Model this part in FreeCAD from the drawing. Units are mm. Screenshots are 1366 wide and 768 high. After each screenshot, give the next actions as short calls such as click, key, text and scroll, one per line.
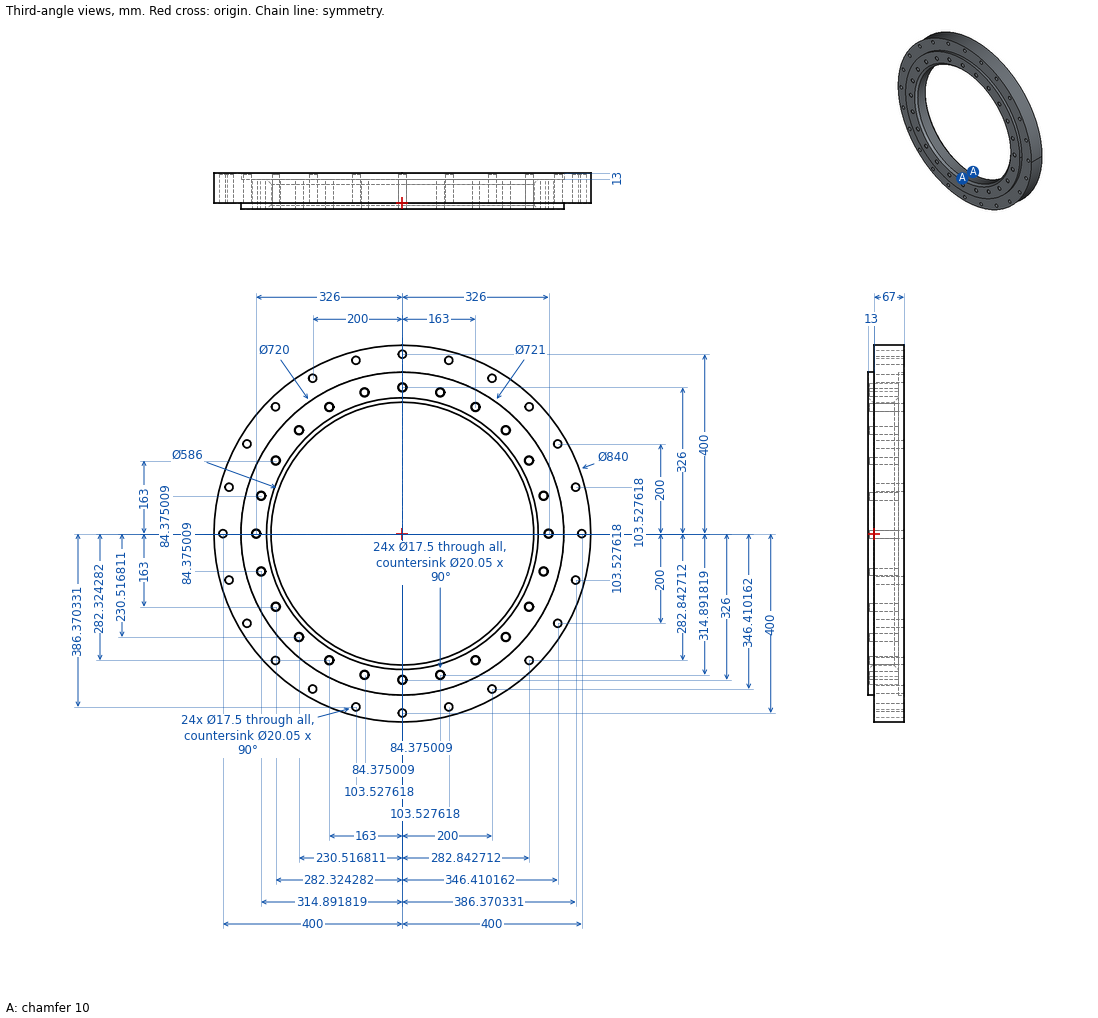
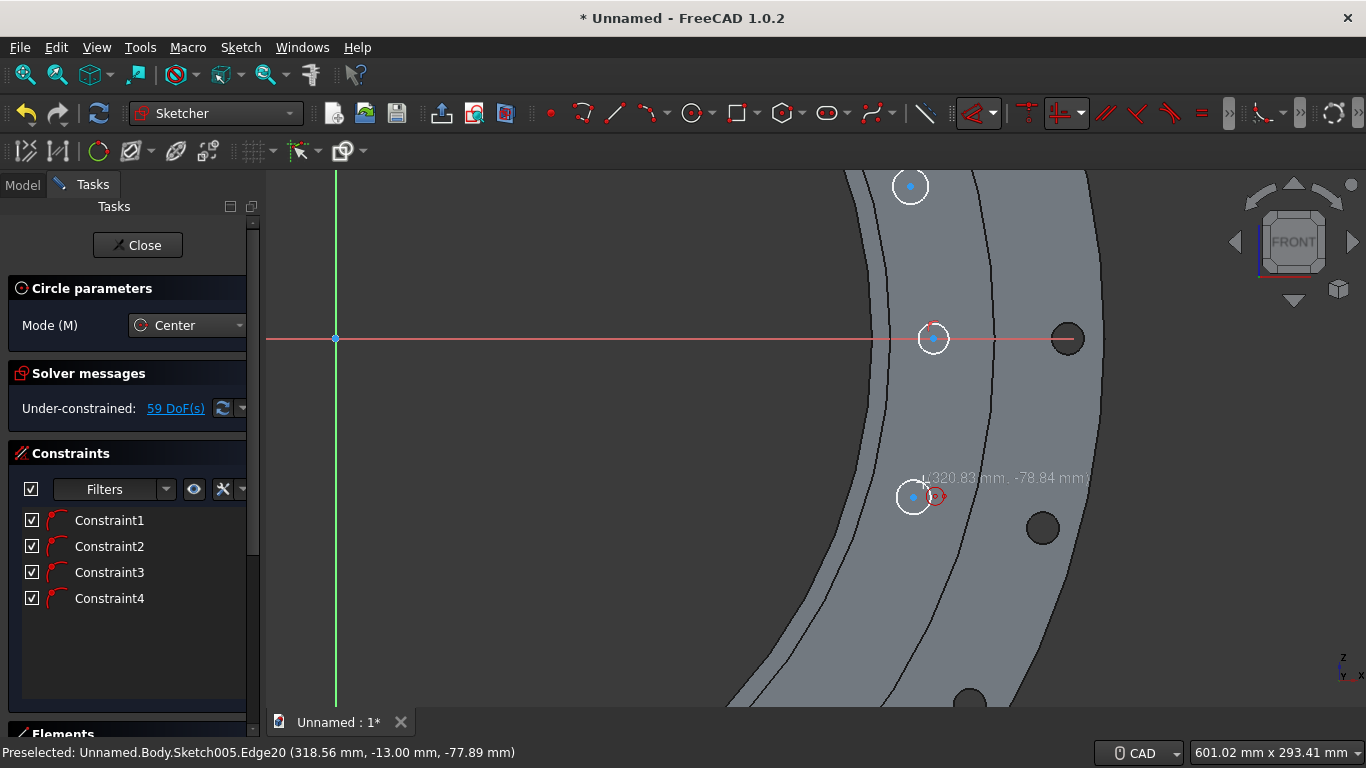
scroll(853, 637, up, 2)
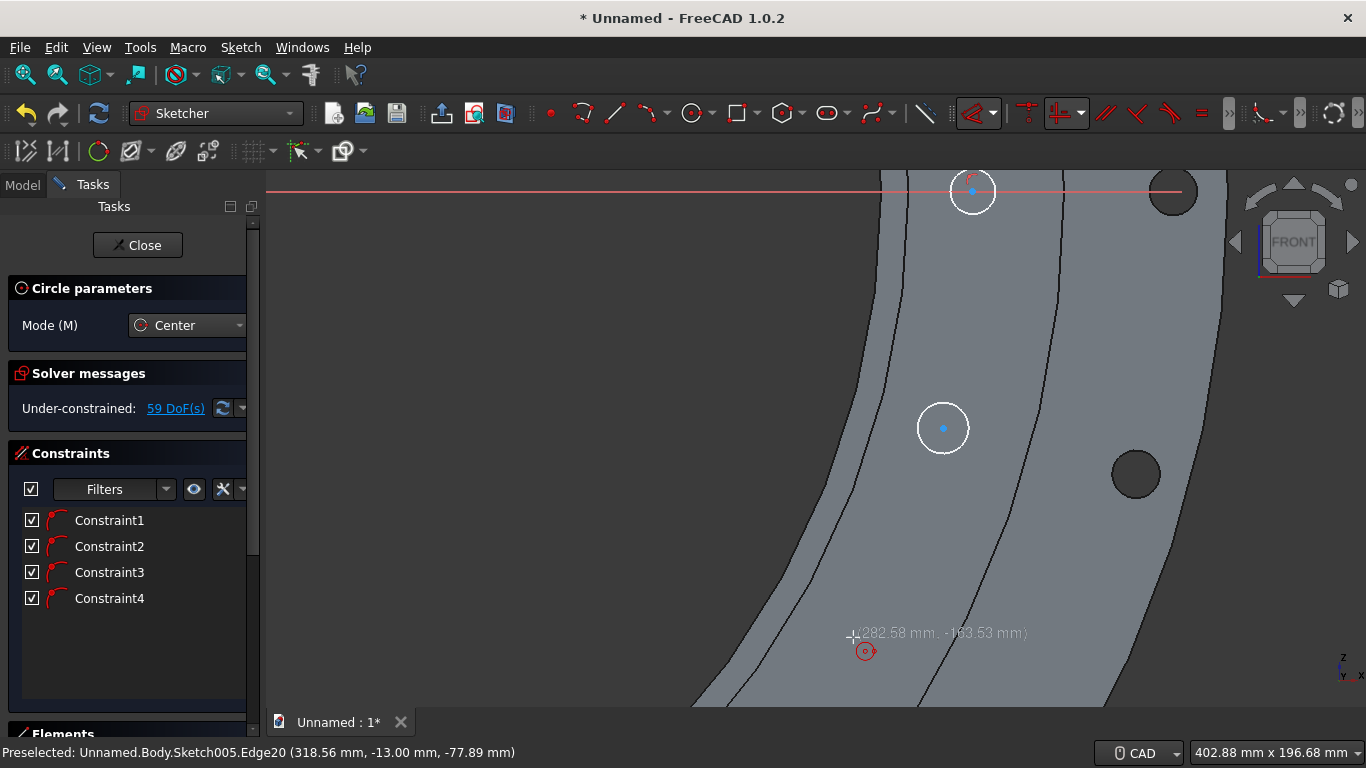
scroll(916, 501, down, 8)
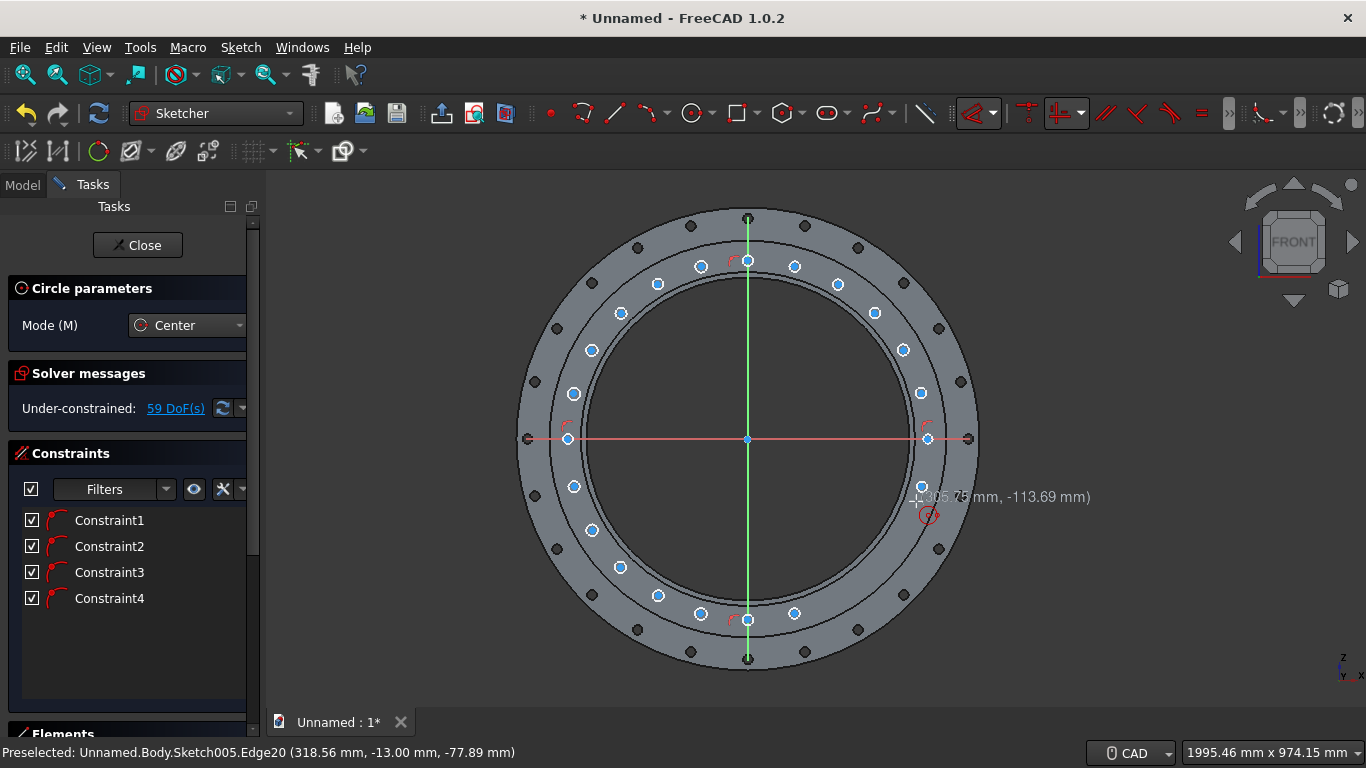
click(904, 529)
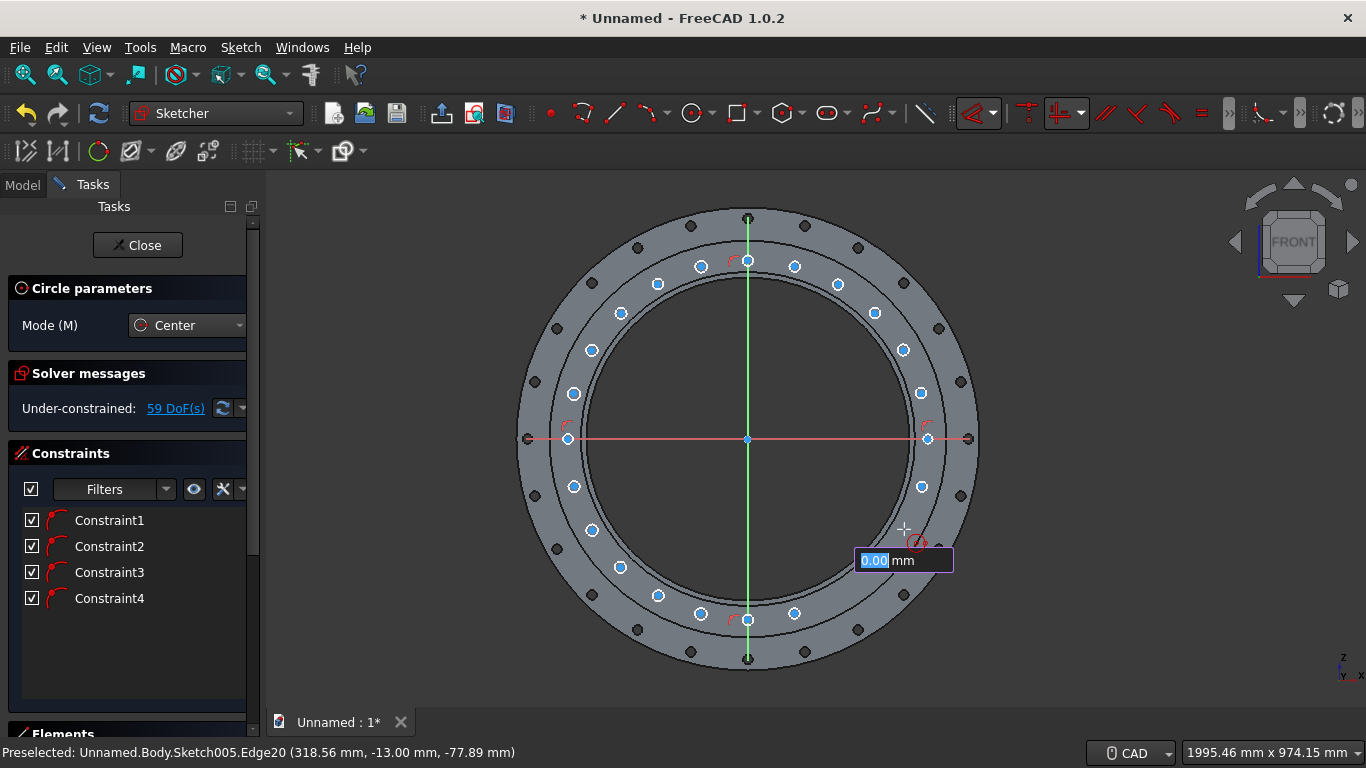
scroll(907, 525, up, 6)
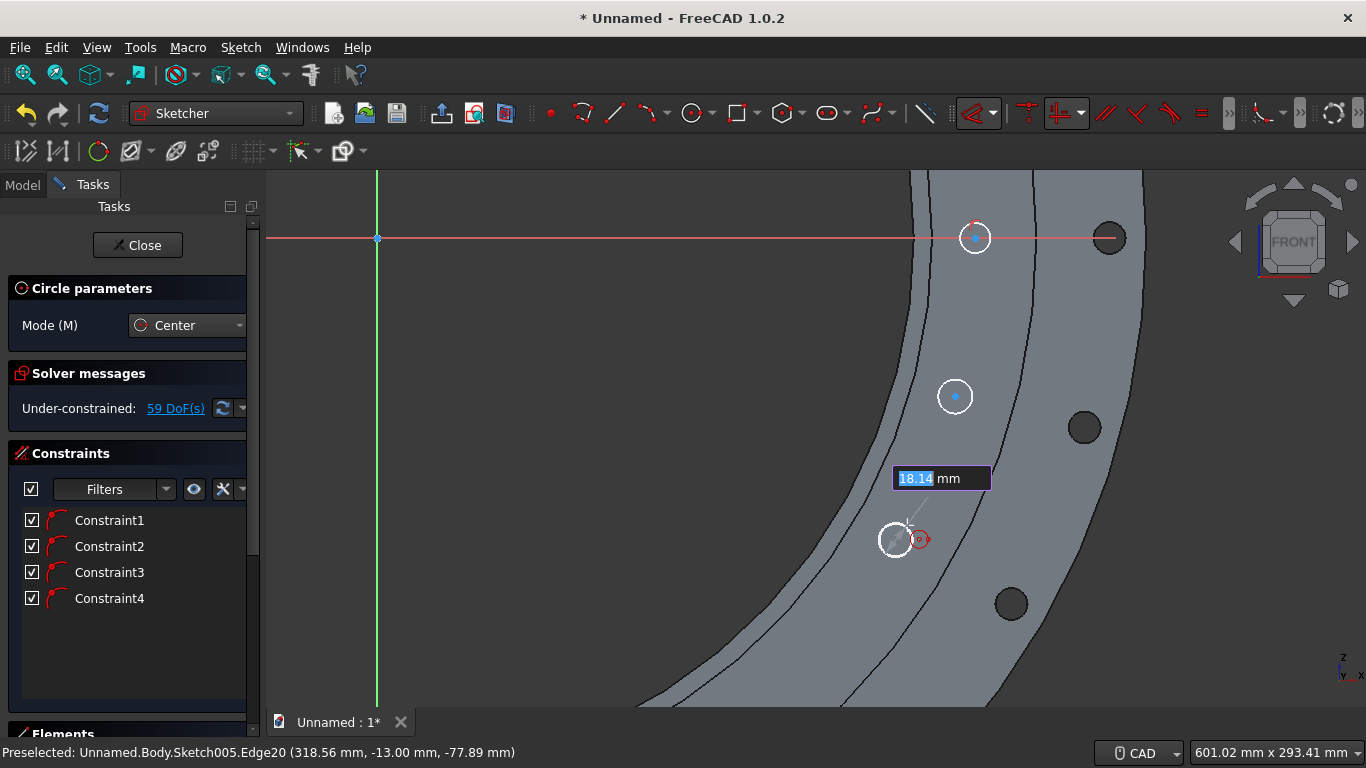
click(906, 525)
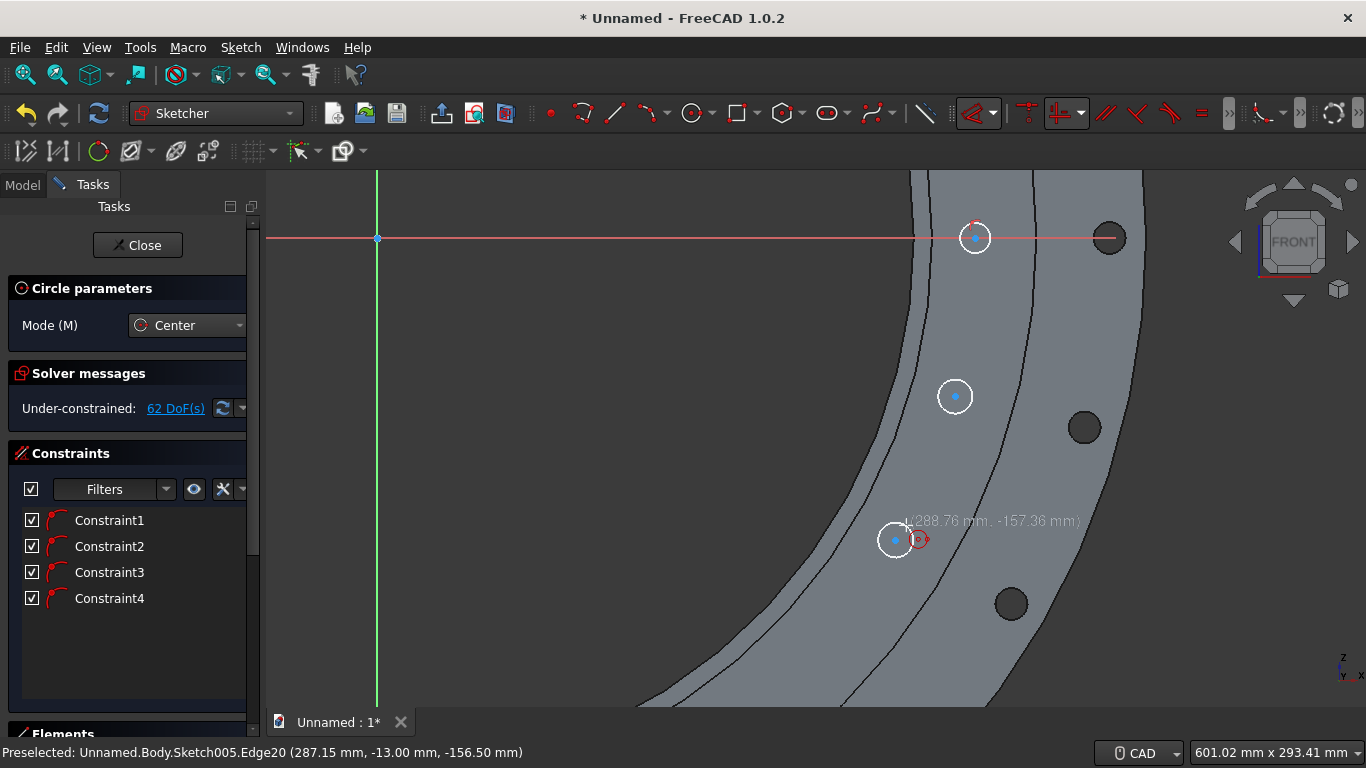
scroll(799, 660, up, 2)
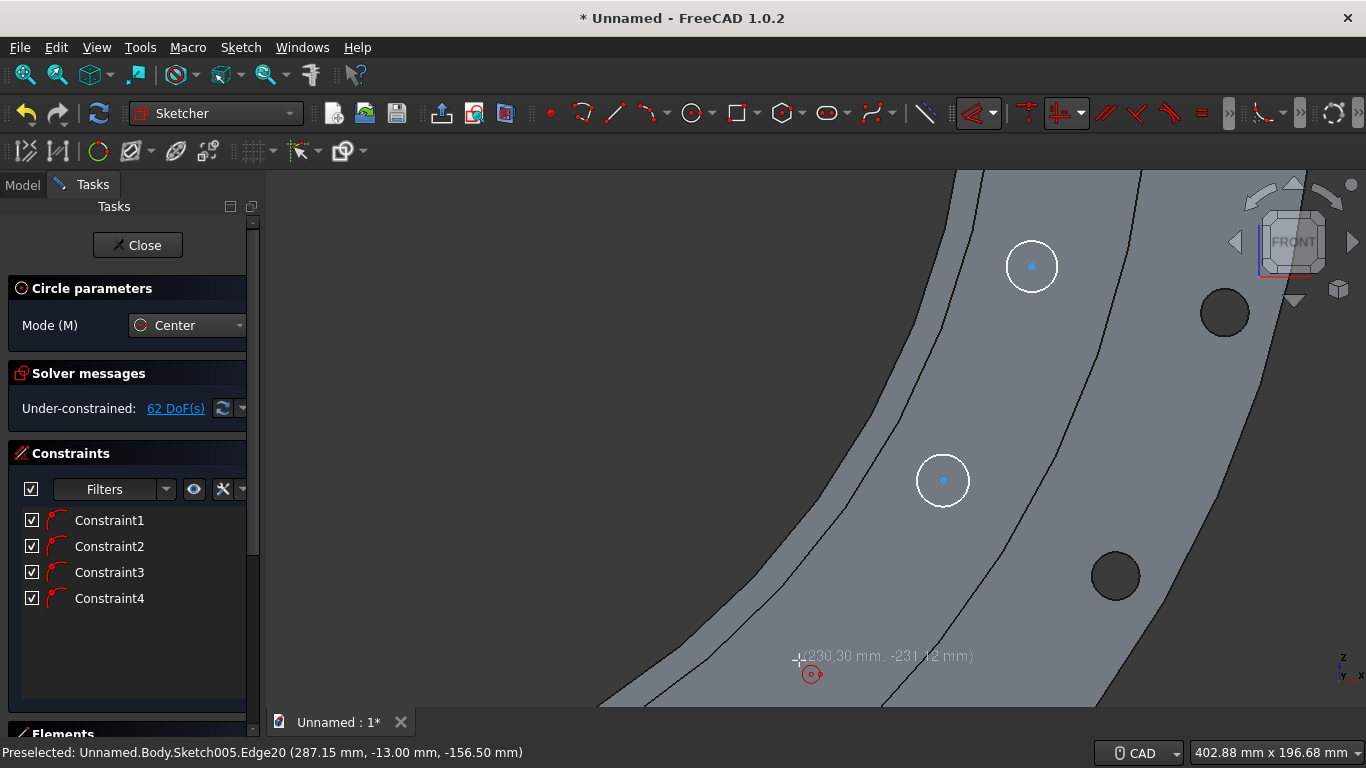
scroll(894, 542, down, 8)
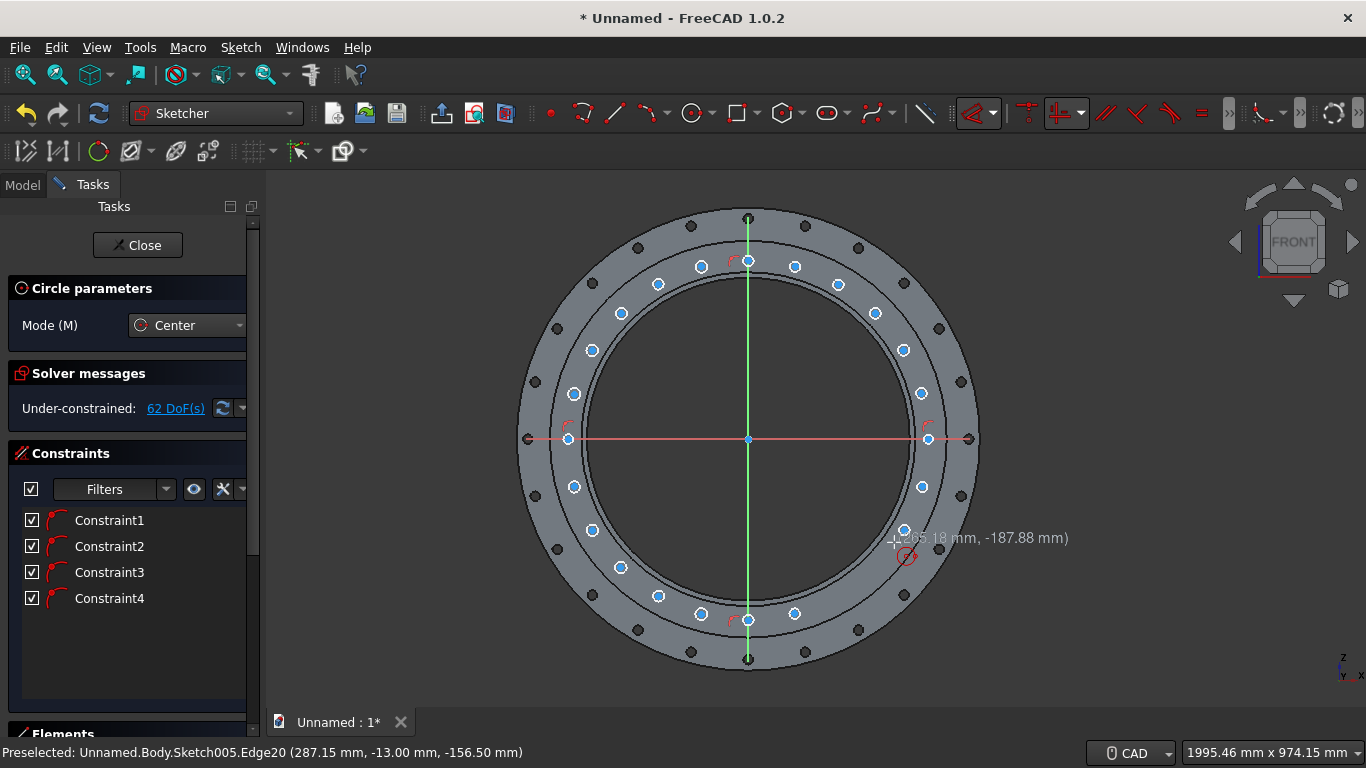
click(875, 566)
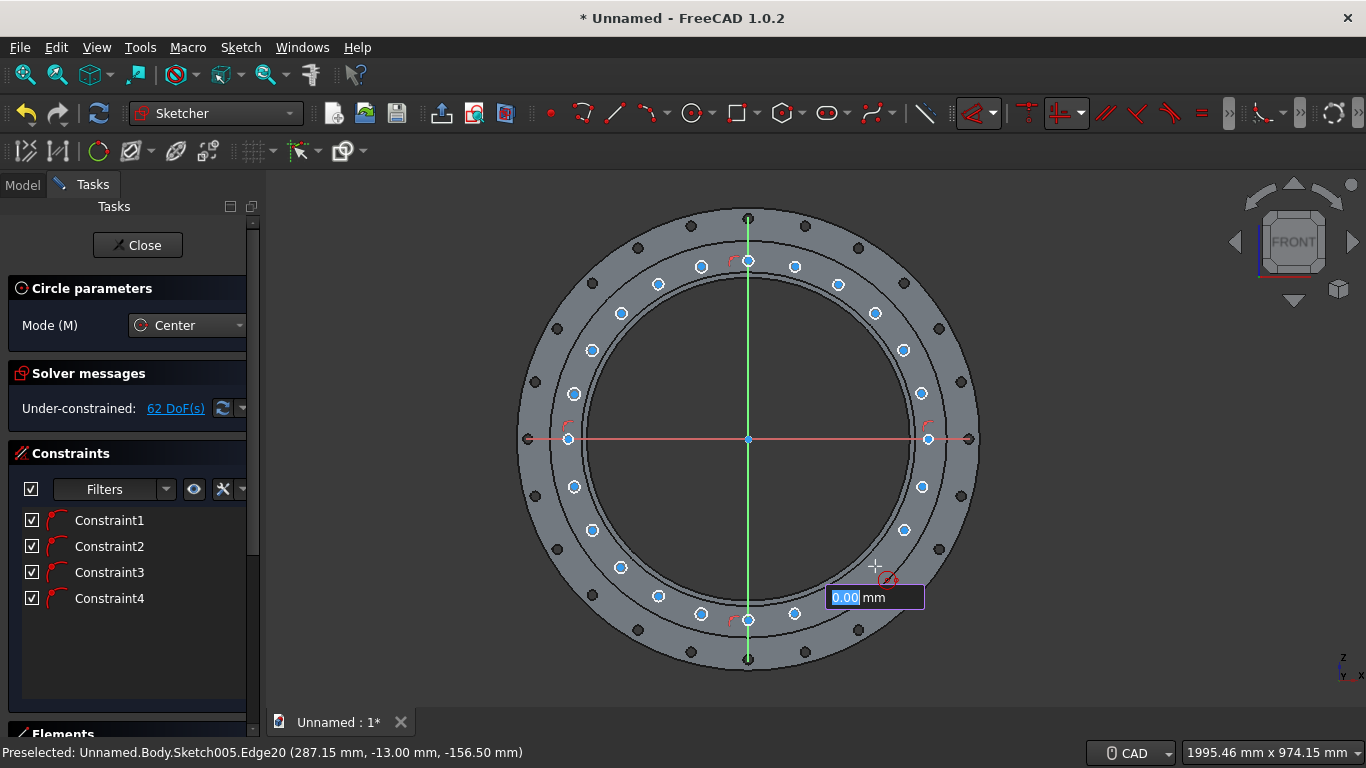
scroll(879, 563, up, 6)